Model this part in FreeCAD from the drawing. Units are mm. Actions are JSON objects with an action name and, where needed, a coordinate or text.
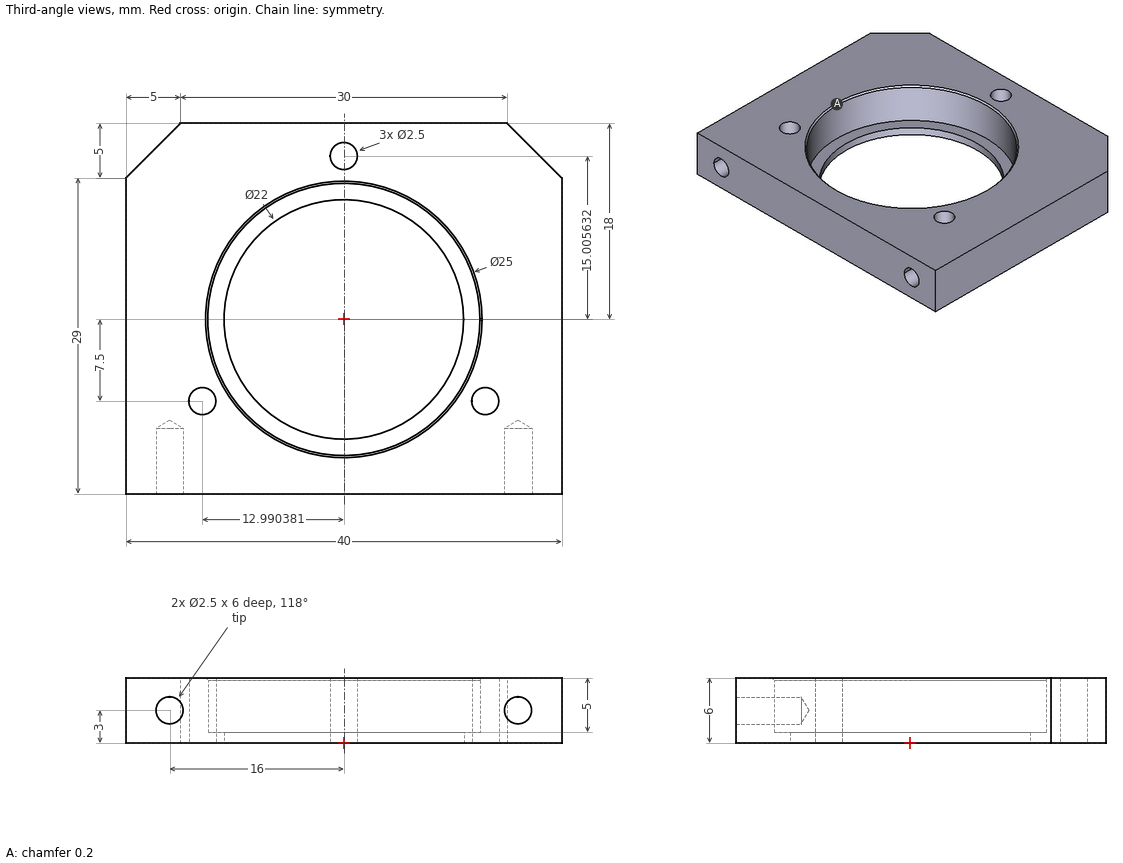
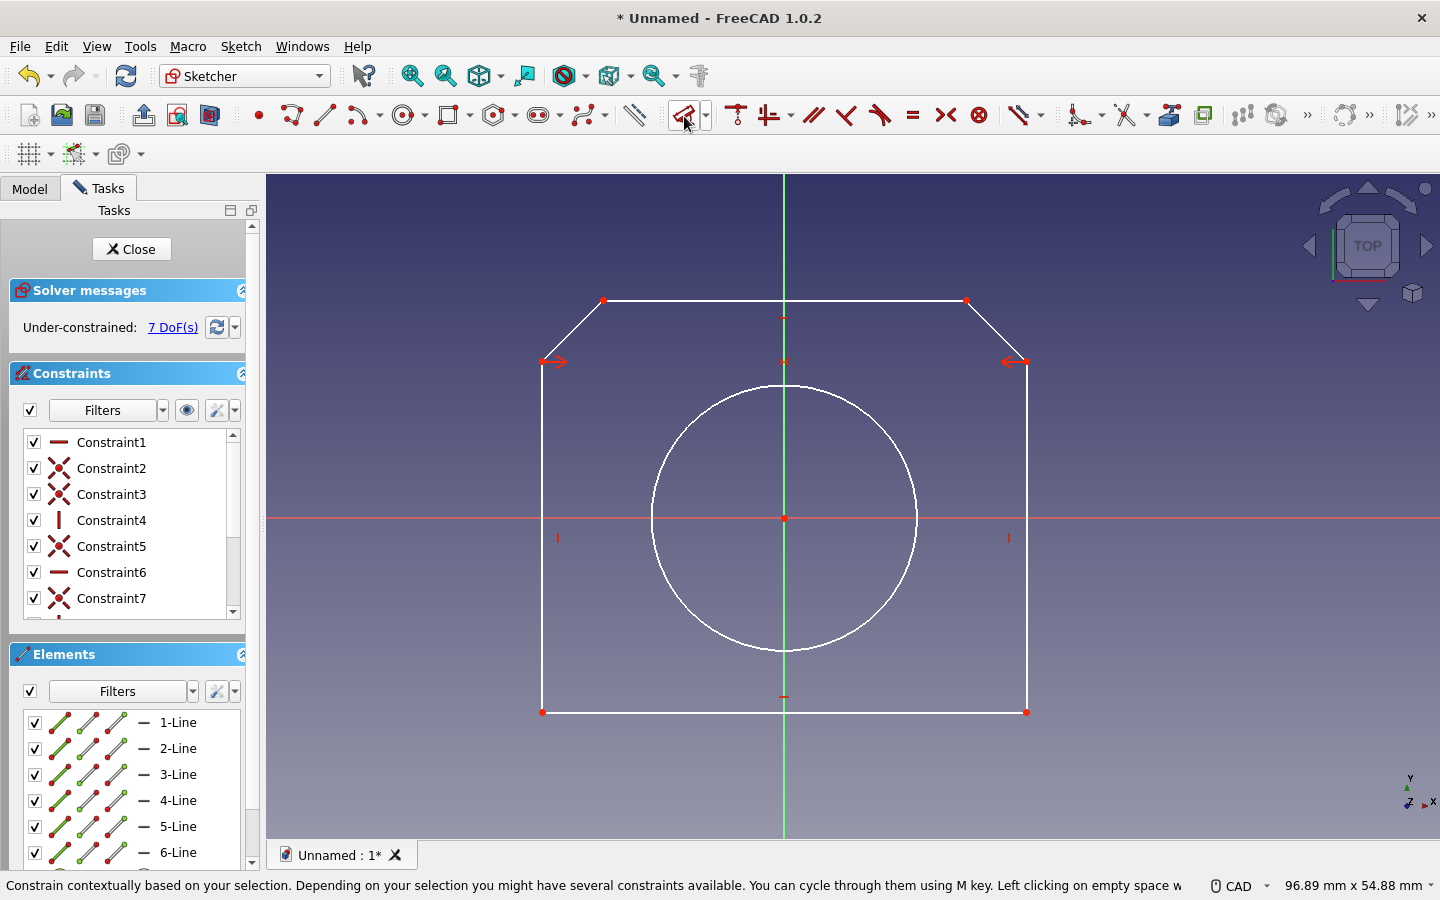
{"action": "left_click", "coordinate": [878, 424]}
{"action": "left_click", "coordinate": [901, 401]}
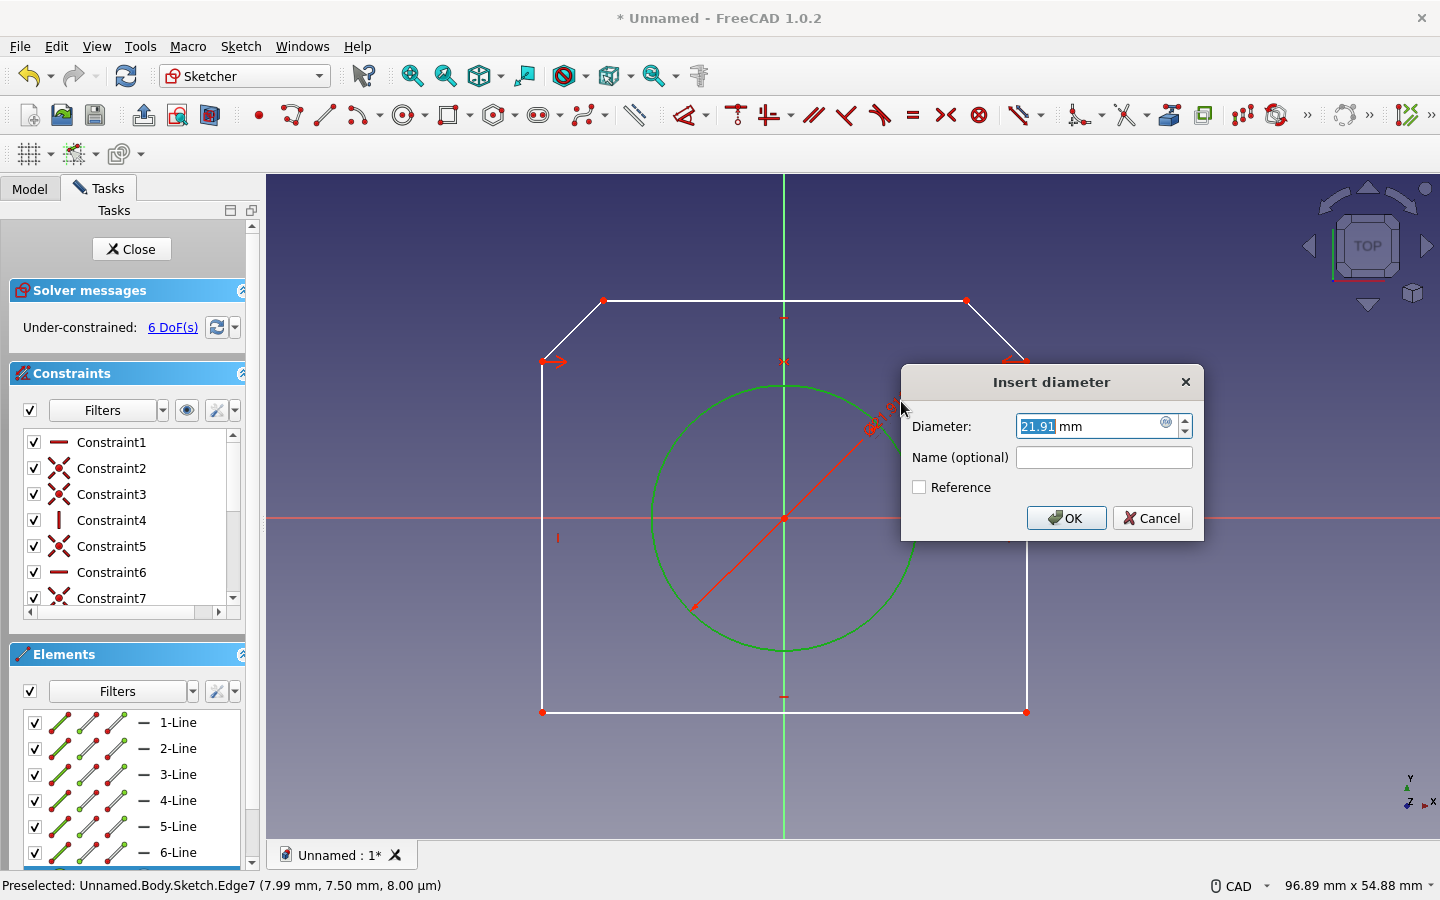
{"action": "type", "text": "22"}
{"action": "key", "text": "Return"}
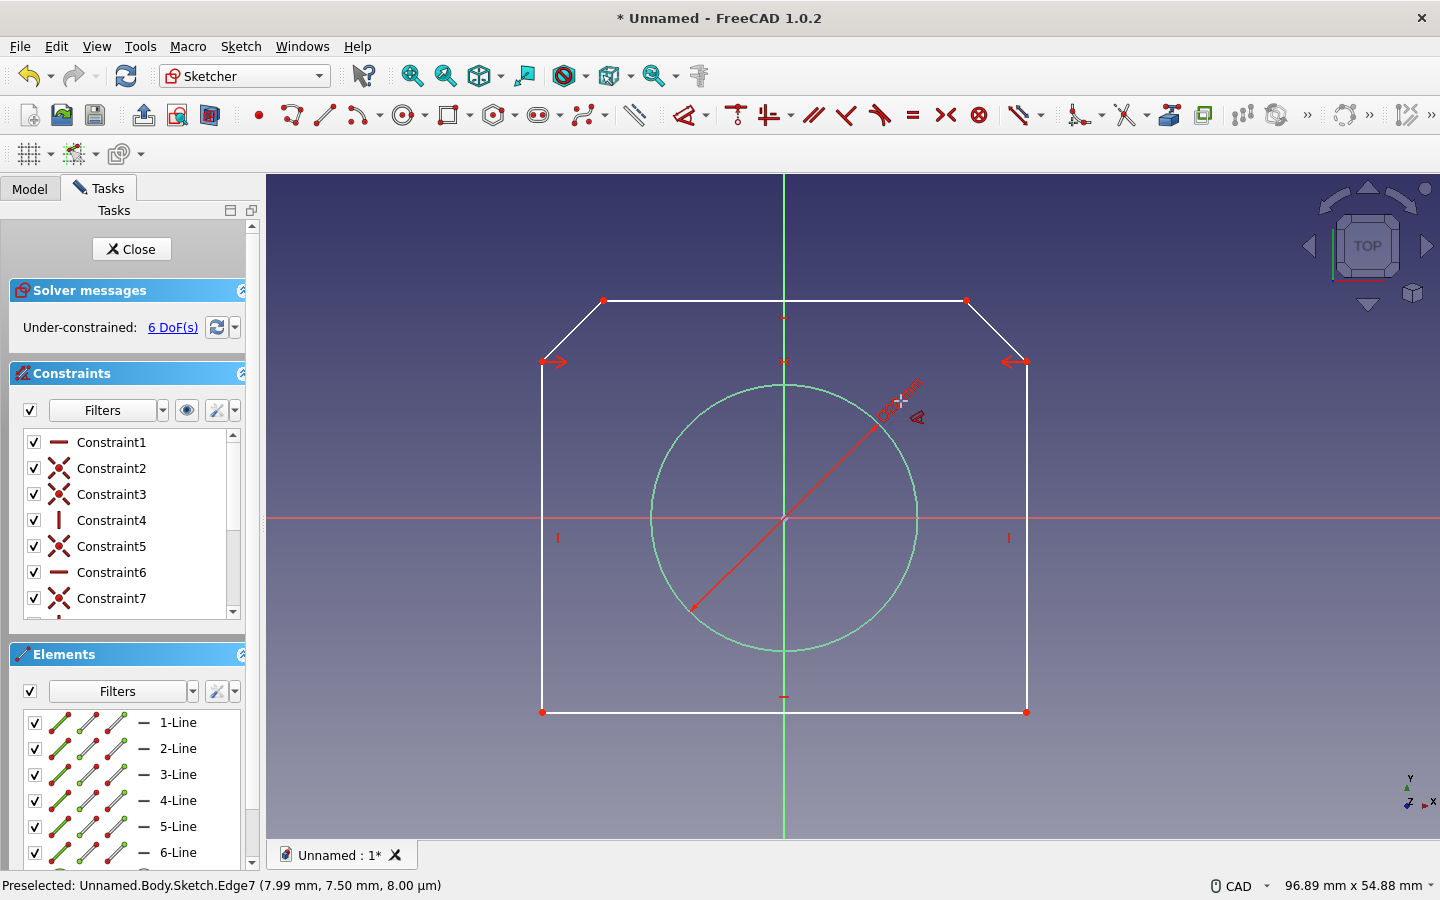
{"action": "left_click", "coordinate": [857, 301]}
{"action": "left_click", "coordinate": [701, 267]}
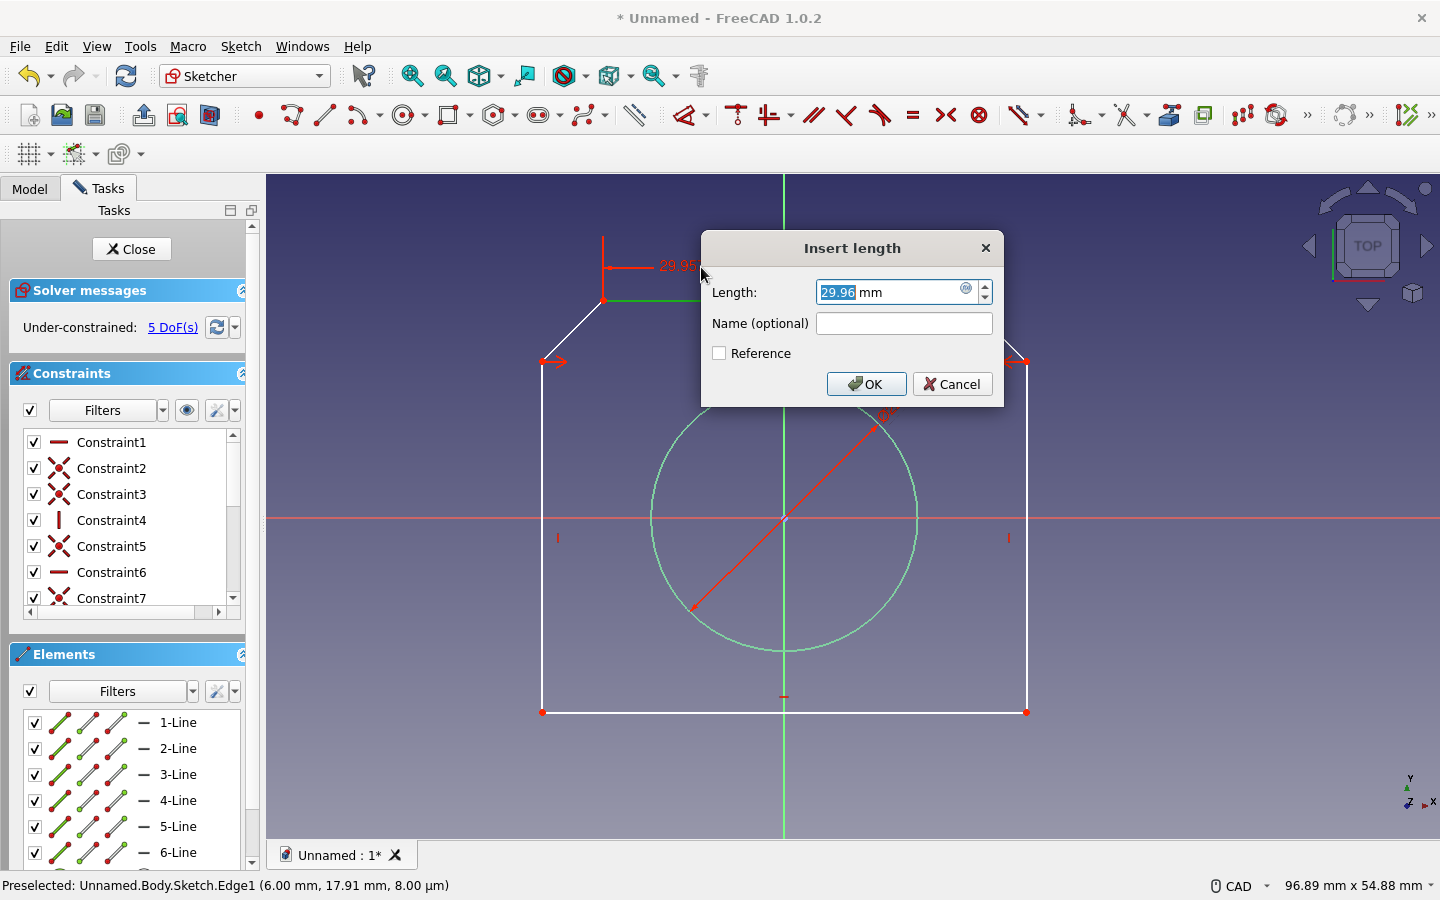
{"action": "type", "text": "30"}
{"action": "key", "text": "Return"}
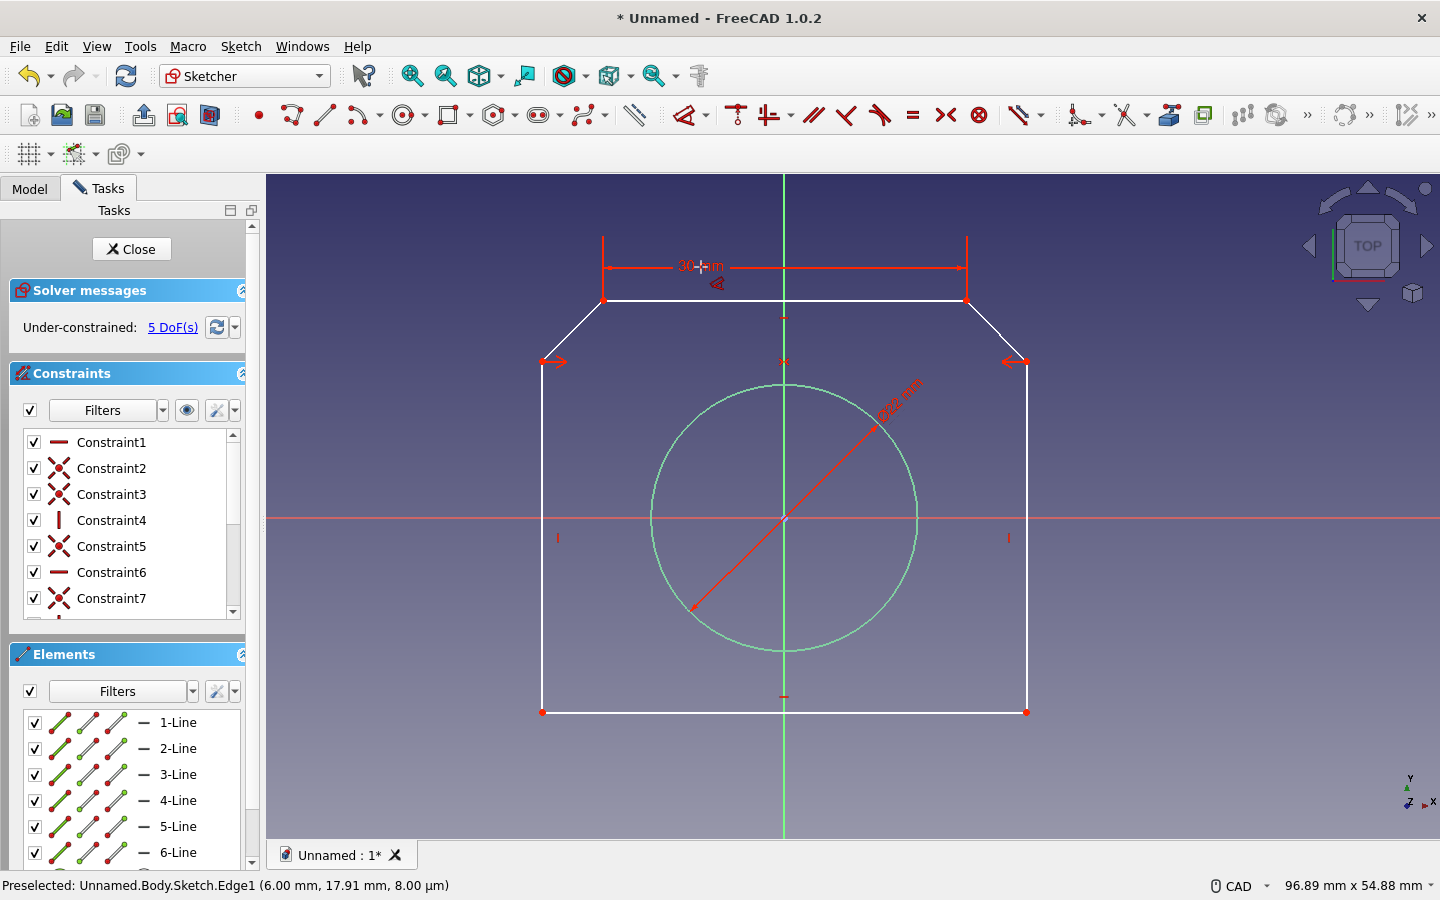
{"action": "left_click", "coordinate": [542, 467]}
{"action": "left_click", "coordinate": [508, 537]}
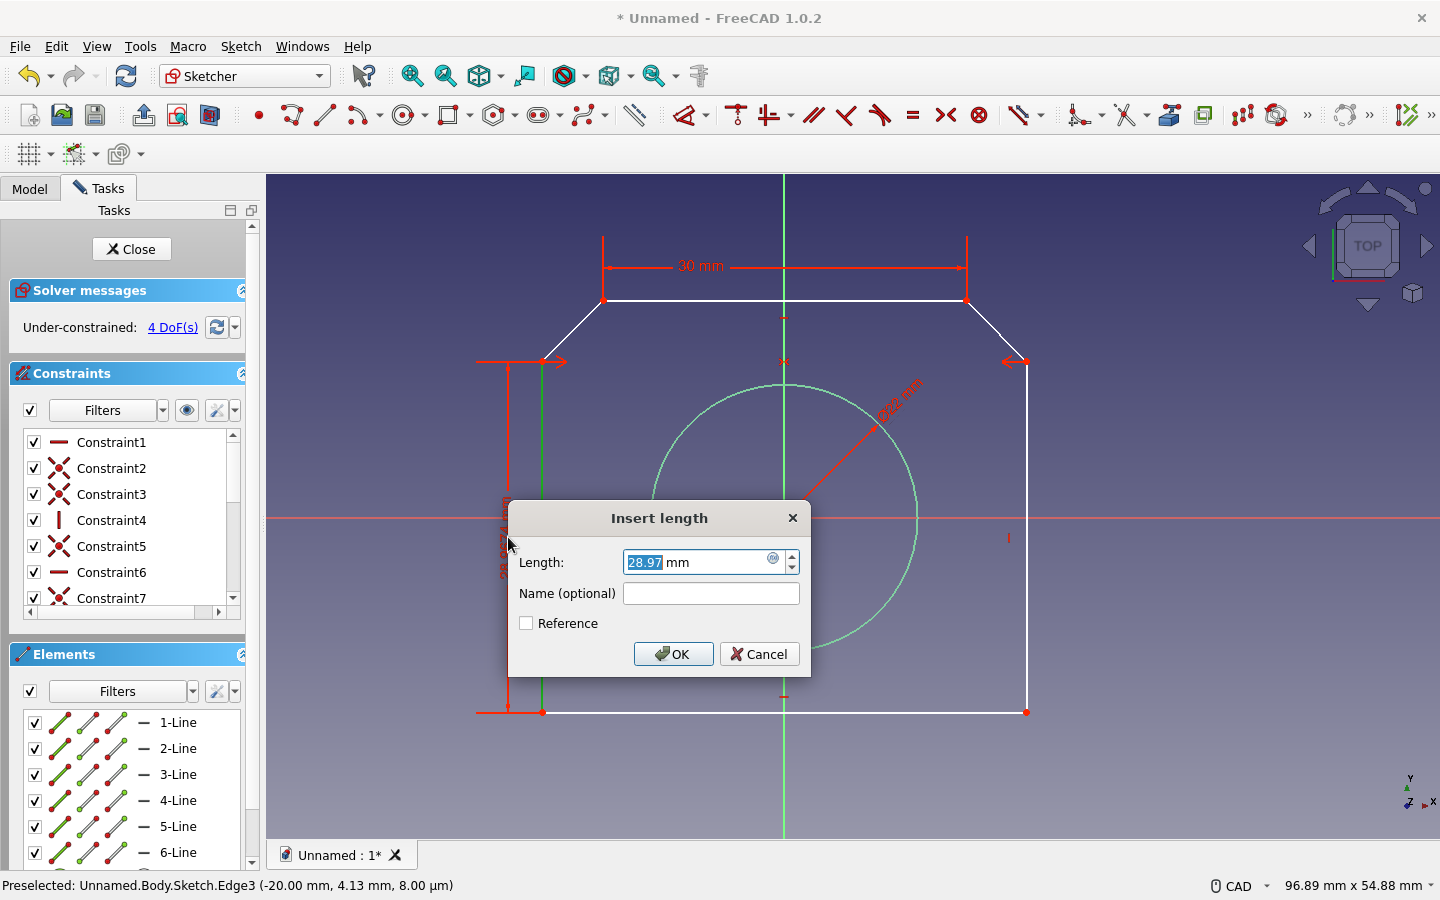
{"action": "type", "text": "29"}
{"action": "key", "text": "Return"}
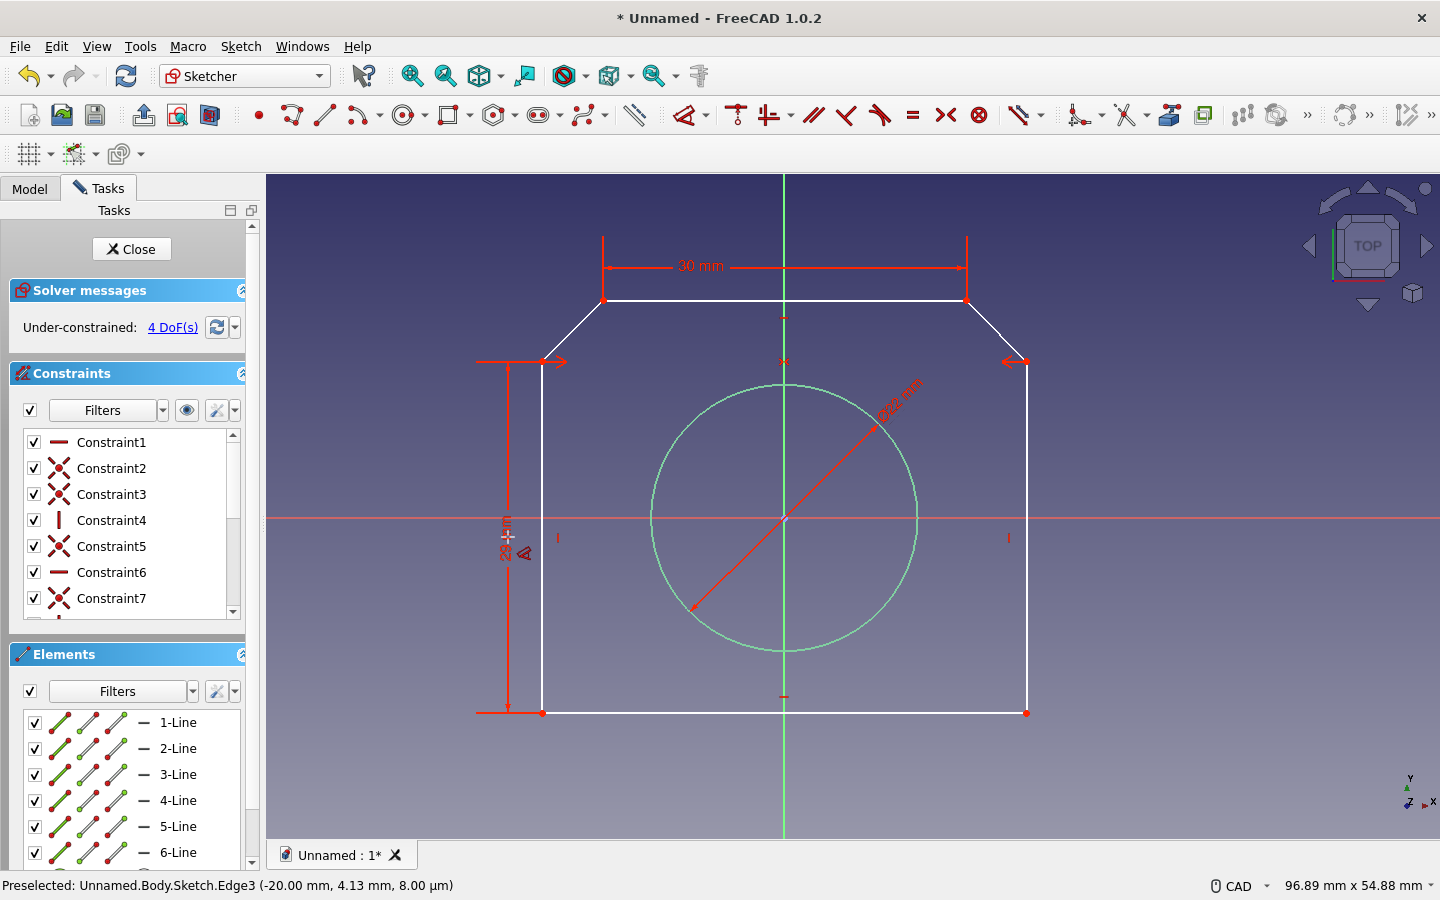
{"action": "left_click", "coordinate": [687, 713]}
{"action": "left_click", "coordinate": [673, 747]}